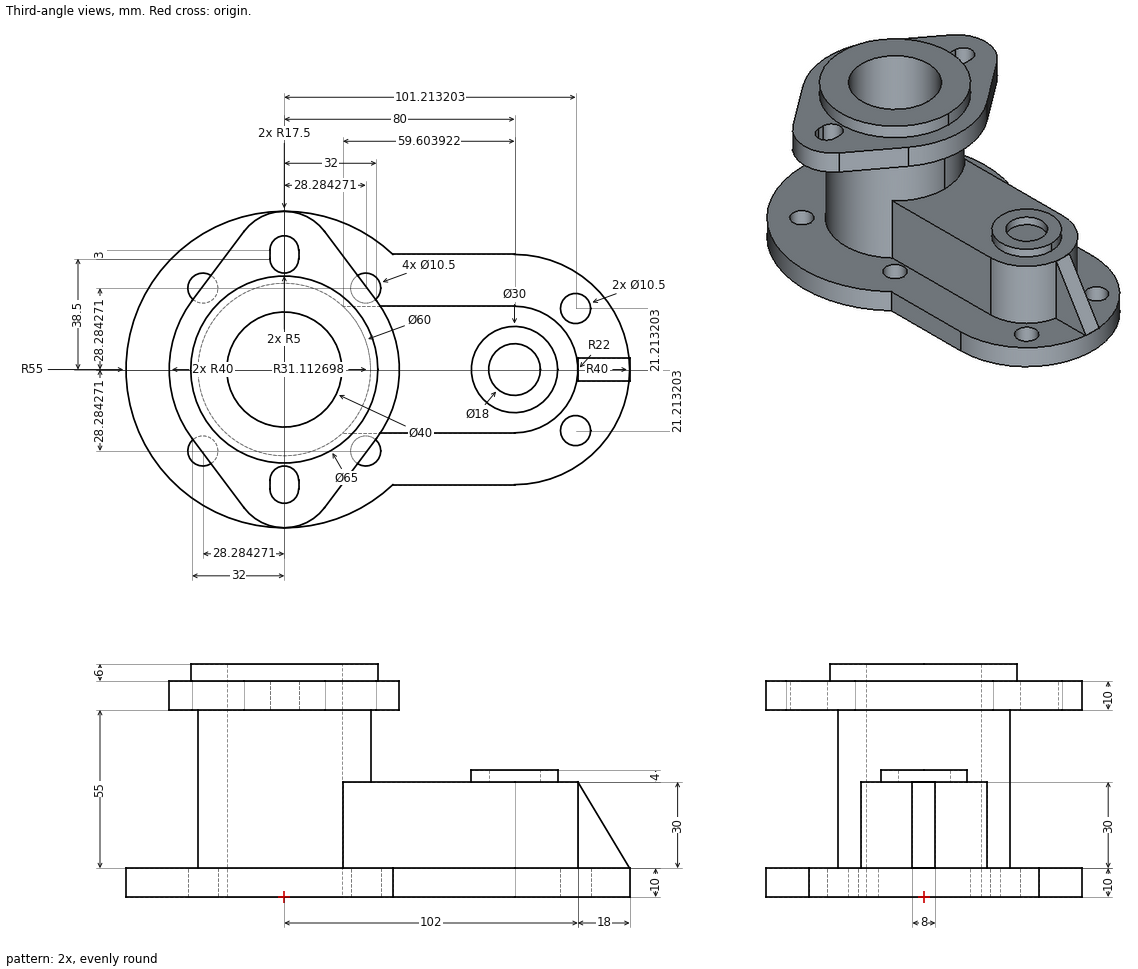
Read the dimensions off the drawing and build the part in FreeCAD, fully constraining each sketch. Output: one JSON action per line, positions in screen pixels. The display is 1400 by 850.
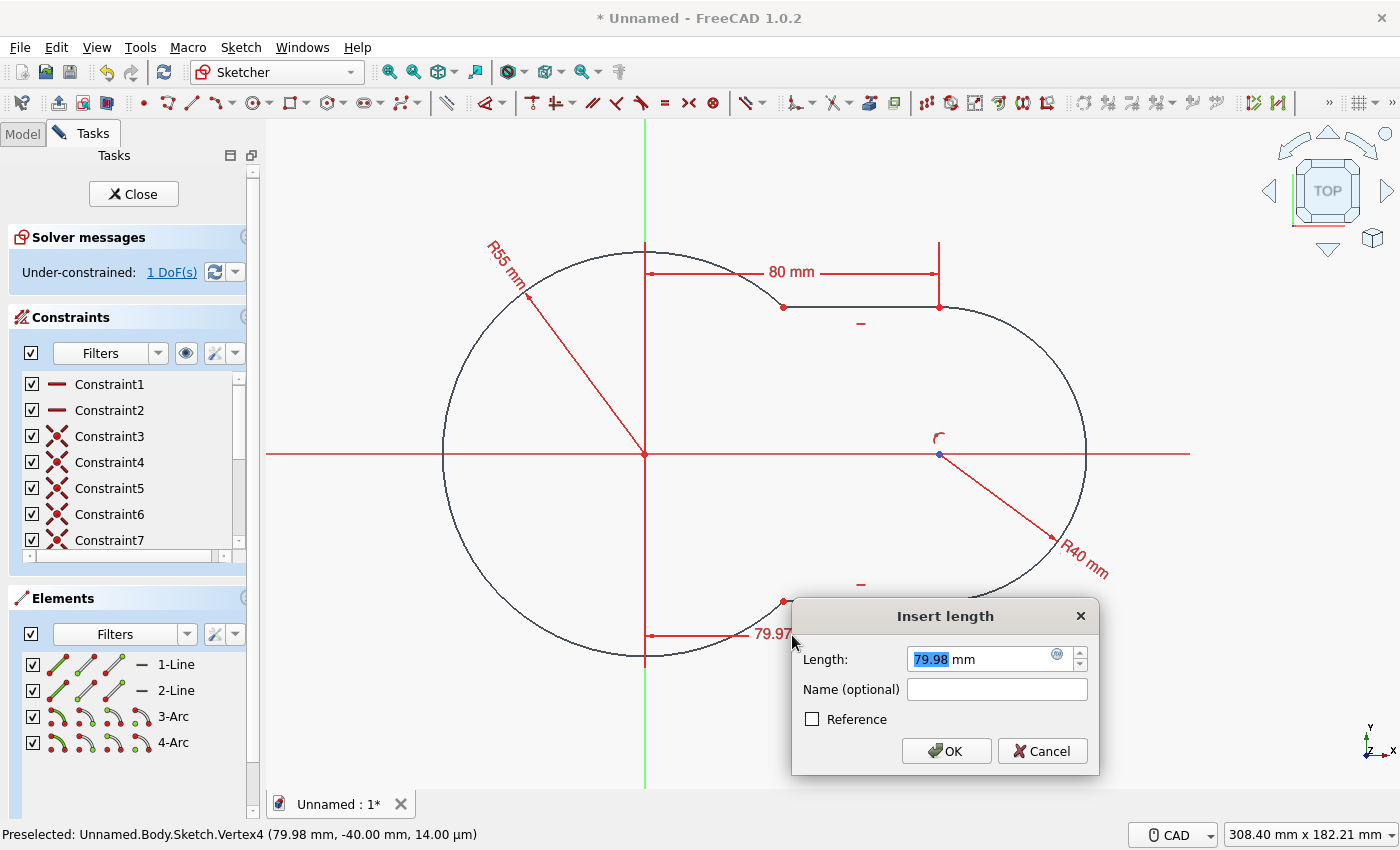
{"action": "type", "text": "80"}
{"action": "key", "text": "Return"}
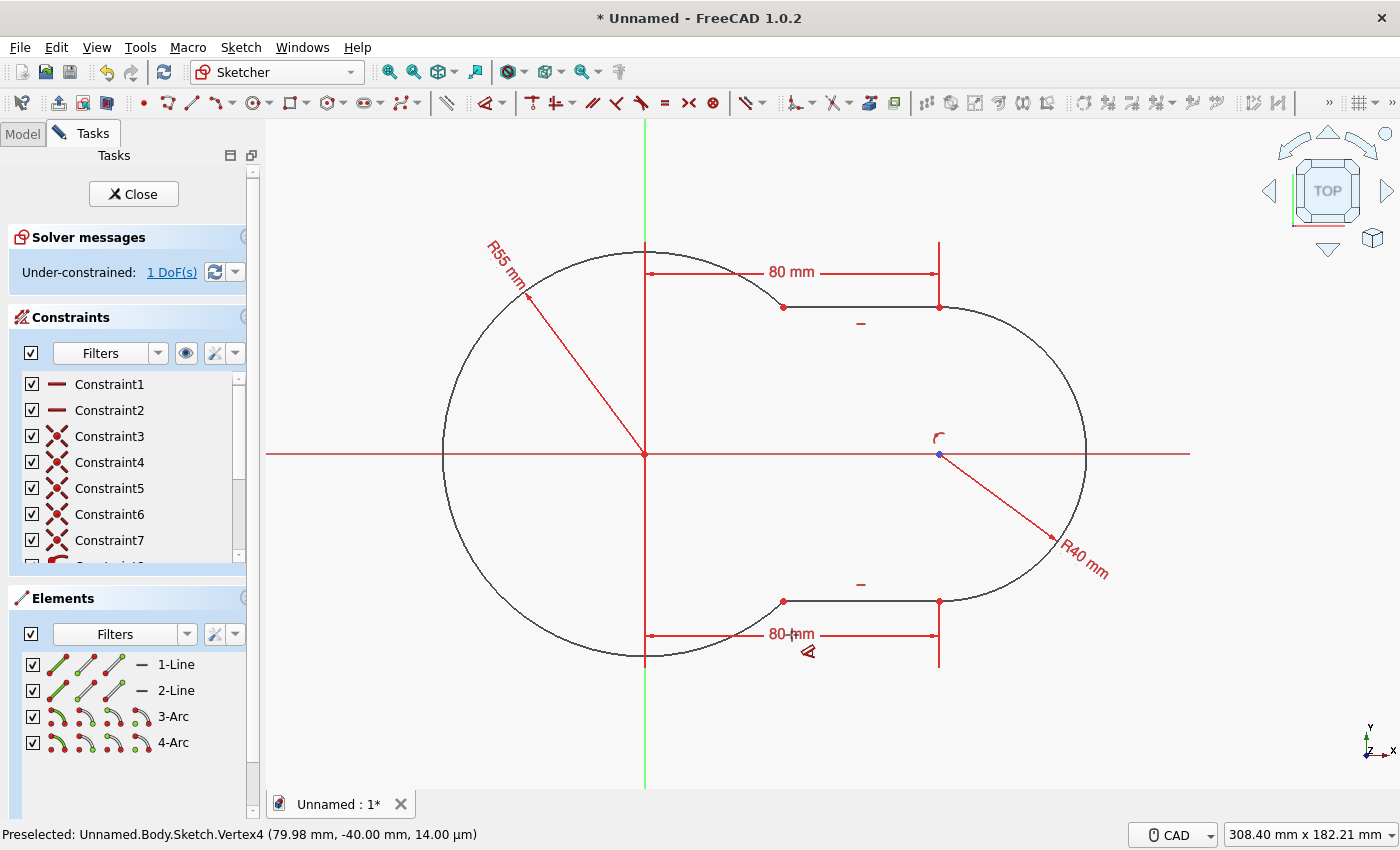
{"action": "left_click", "coordinate": [939, 454]}
{"action": "left_click", "coordinate": [792, 488]}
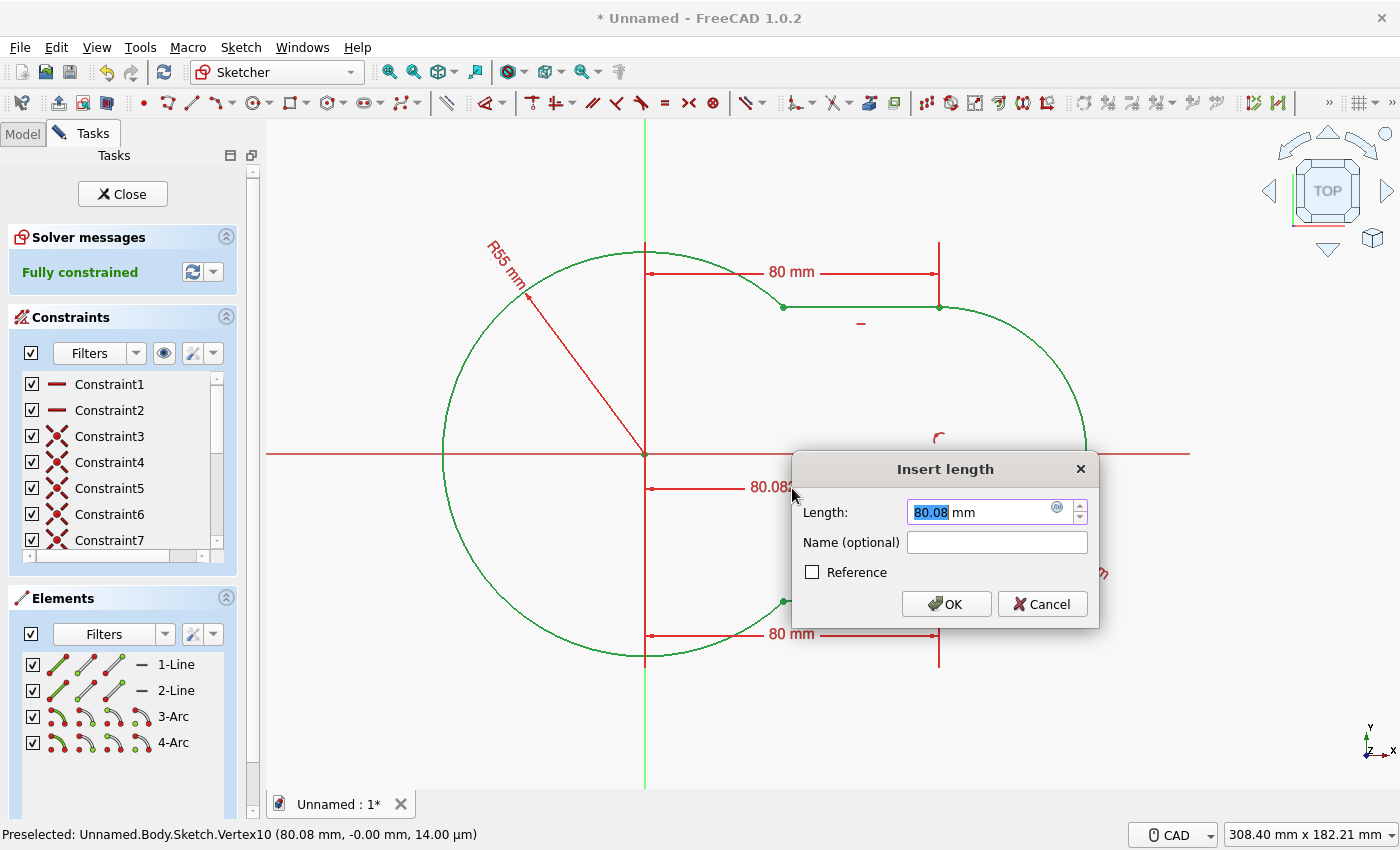
{"action": "type", "text": "80"}
{"action": "key", "text": "Return"}
{"action": "key", "text": "Escape"}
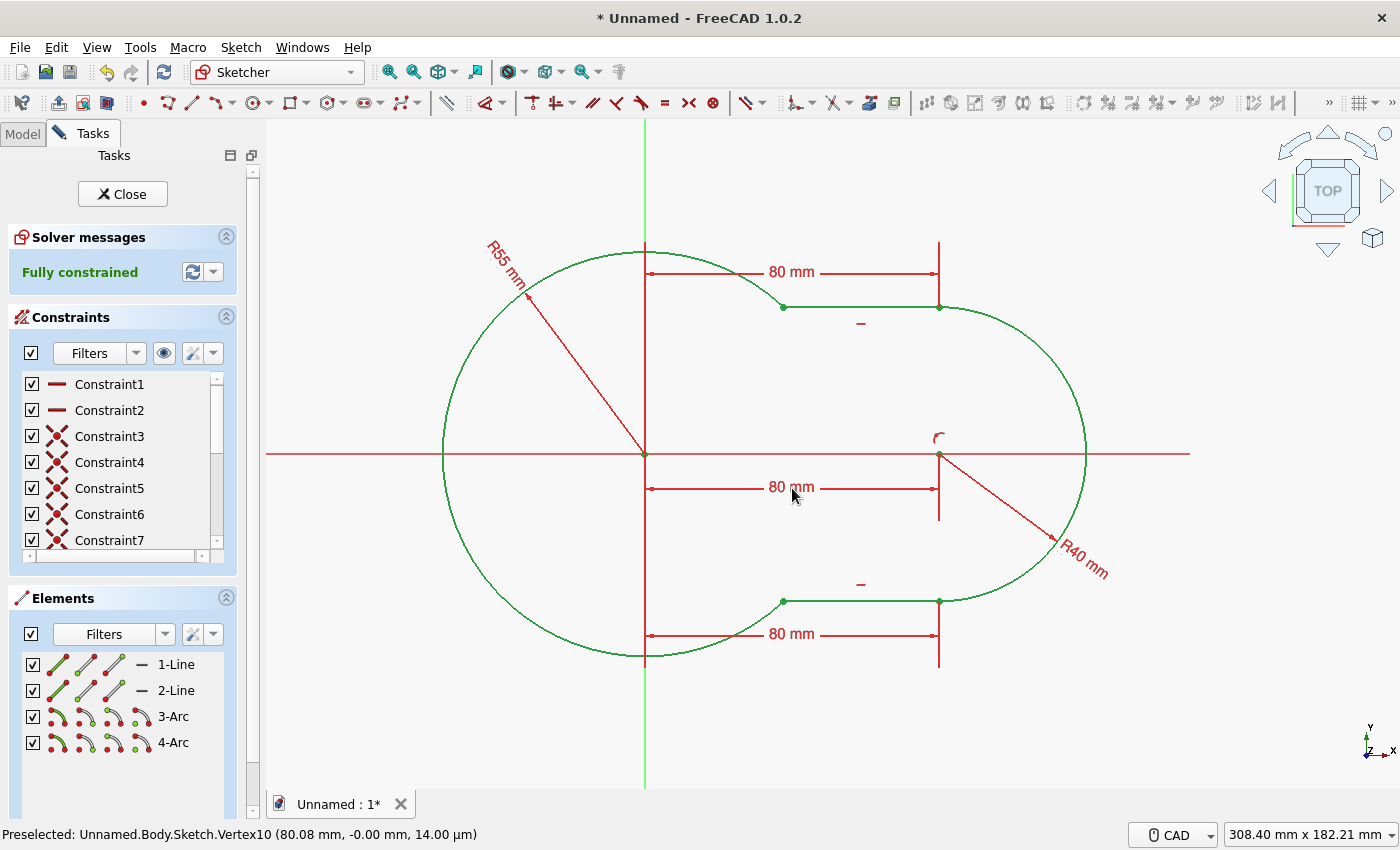
{"action": "left_click", "coordinate": [123, 194]}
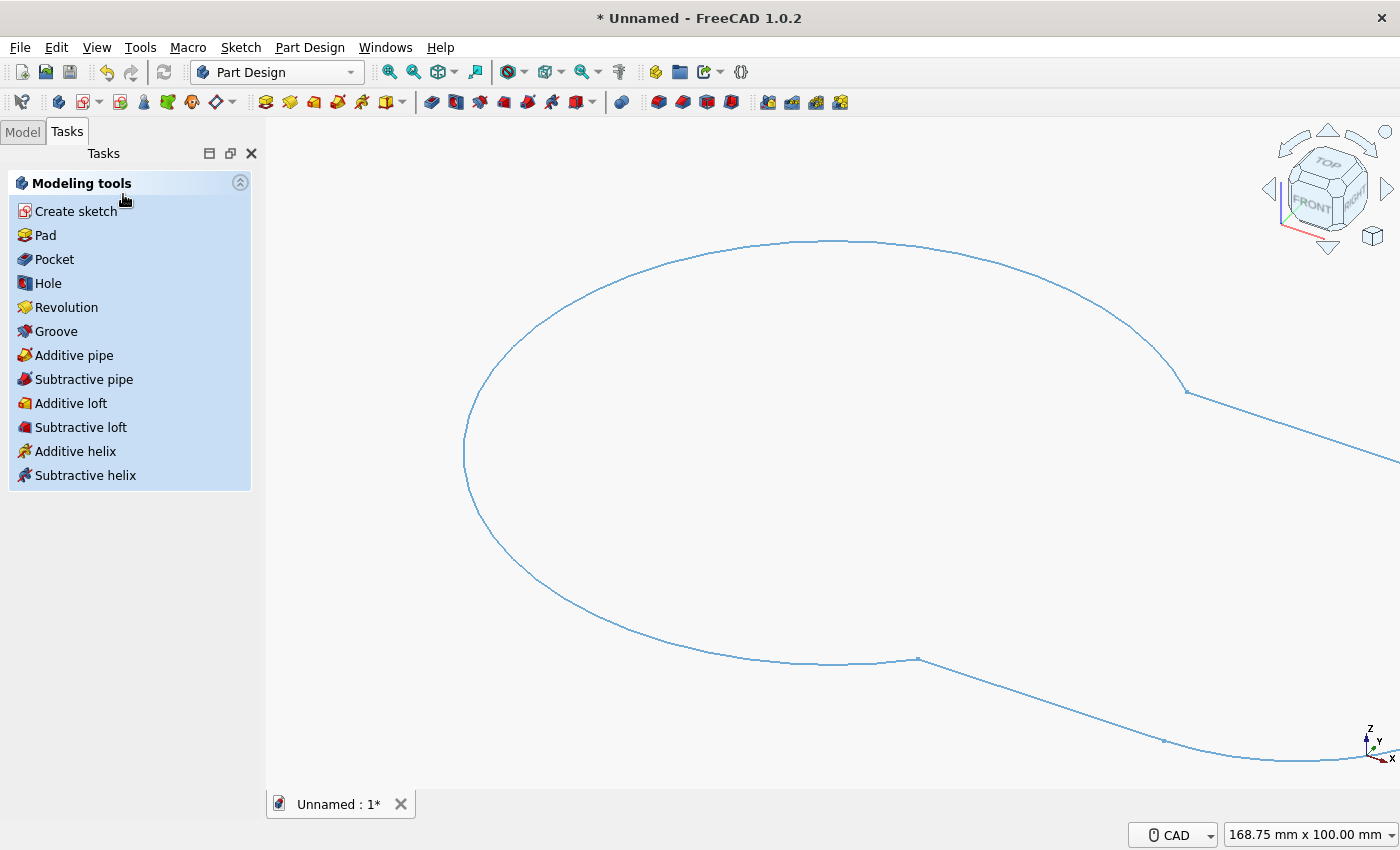
{"action": "left_click", "coordinate": [266, 102]}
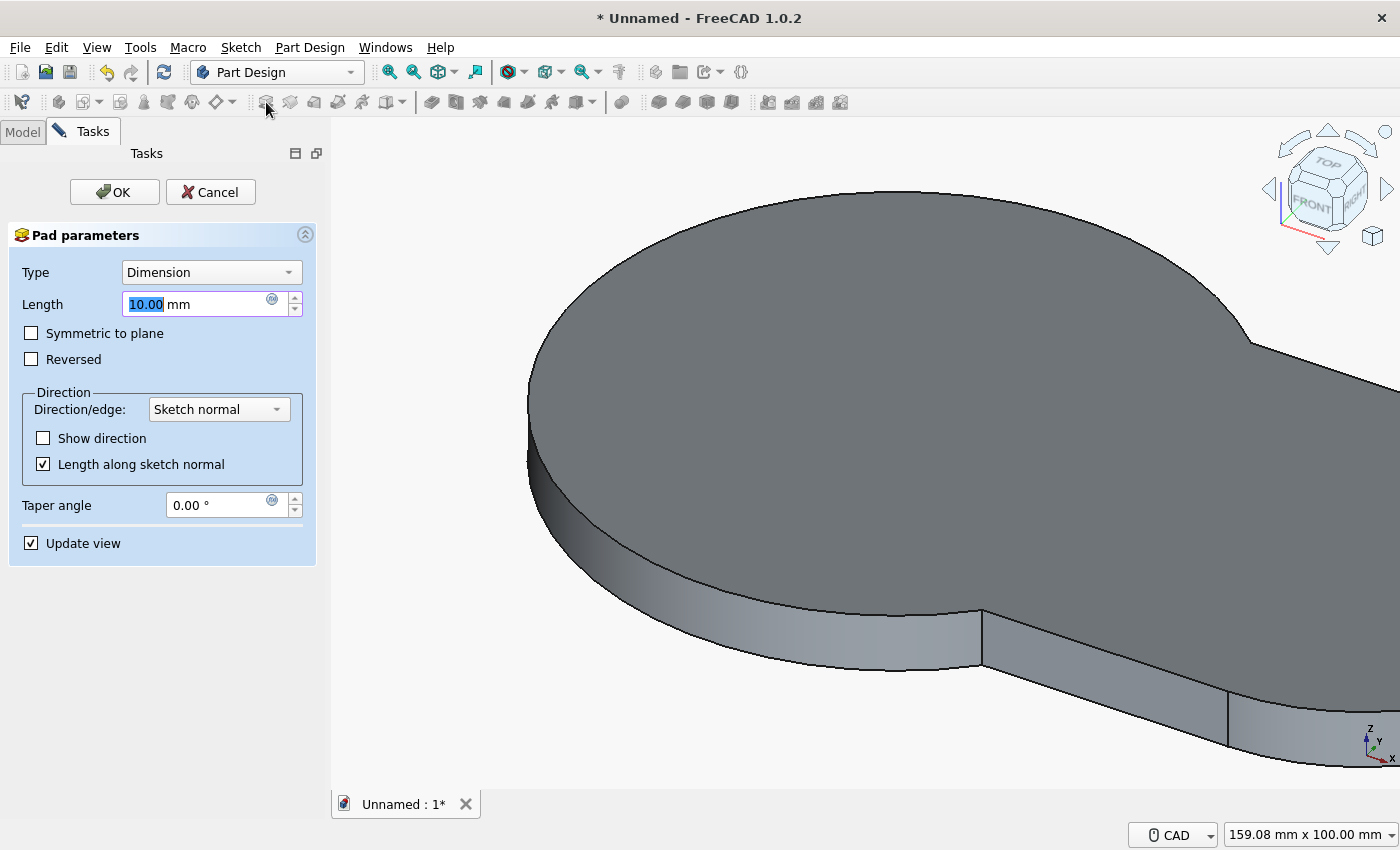
{"action": "type", "text": "10"}
{"action": "key", "text": "Tab"}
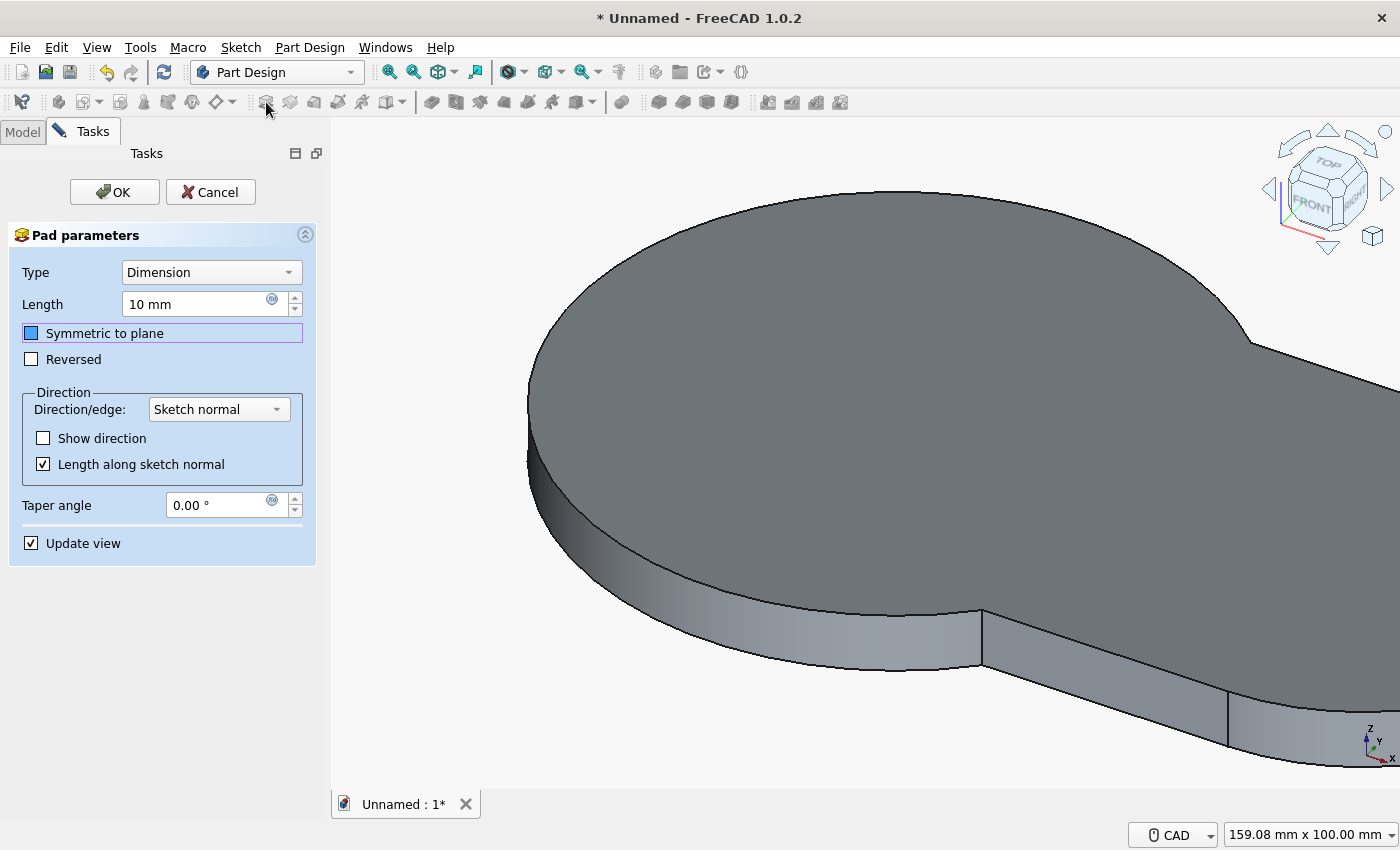
{"action": "left_click", "coordinate": [115, 192]}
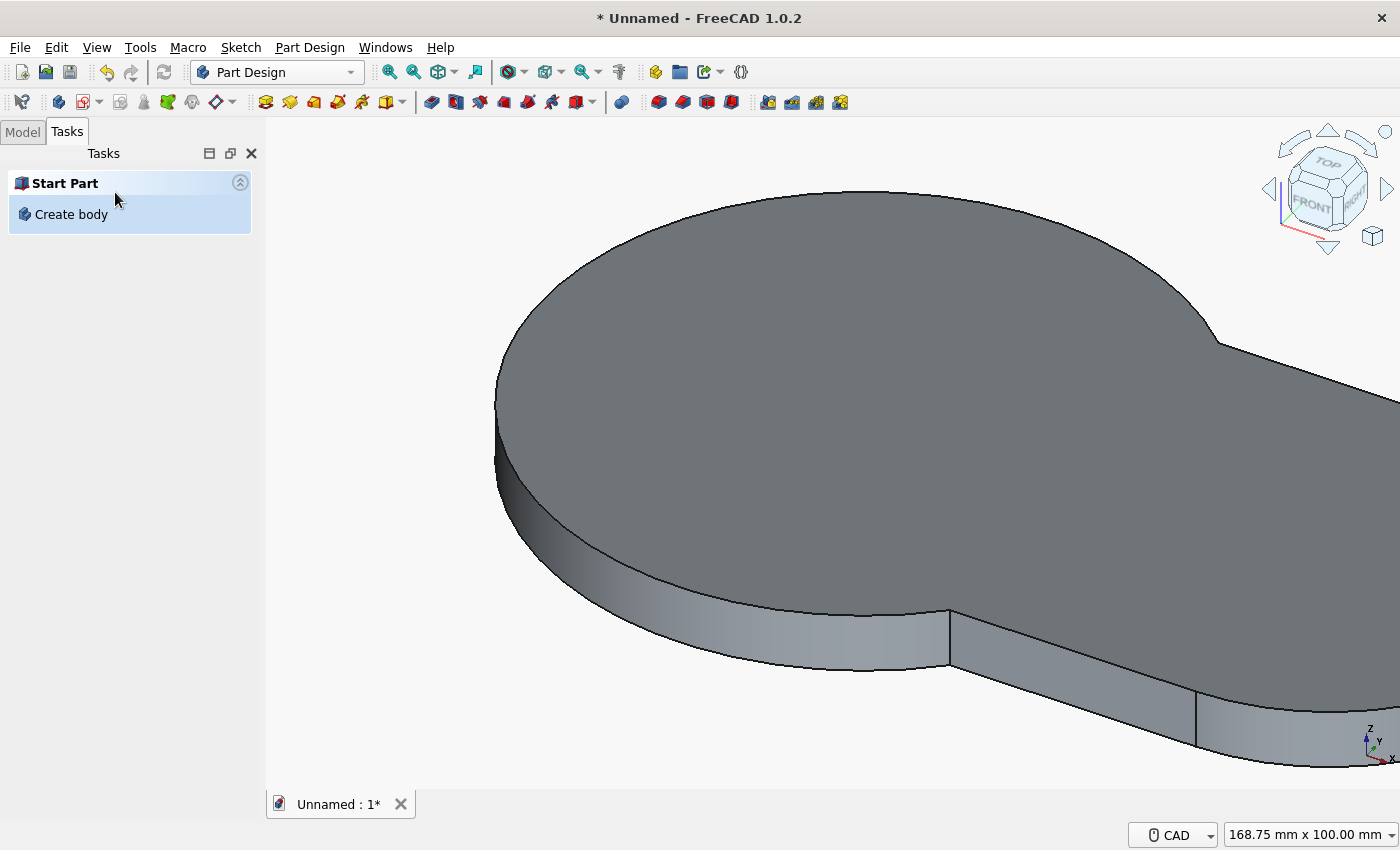
{"action": "key", "text": "v f"}